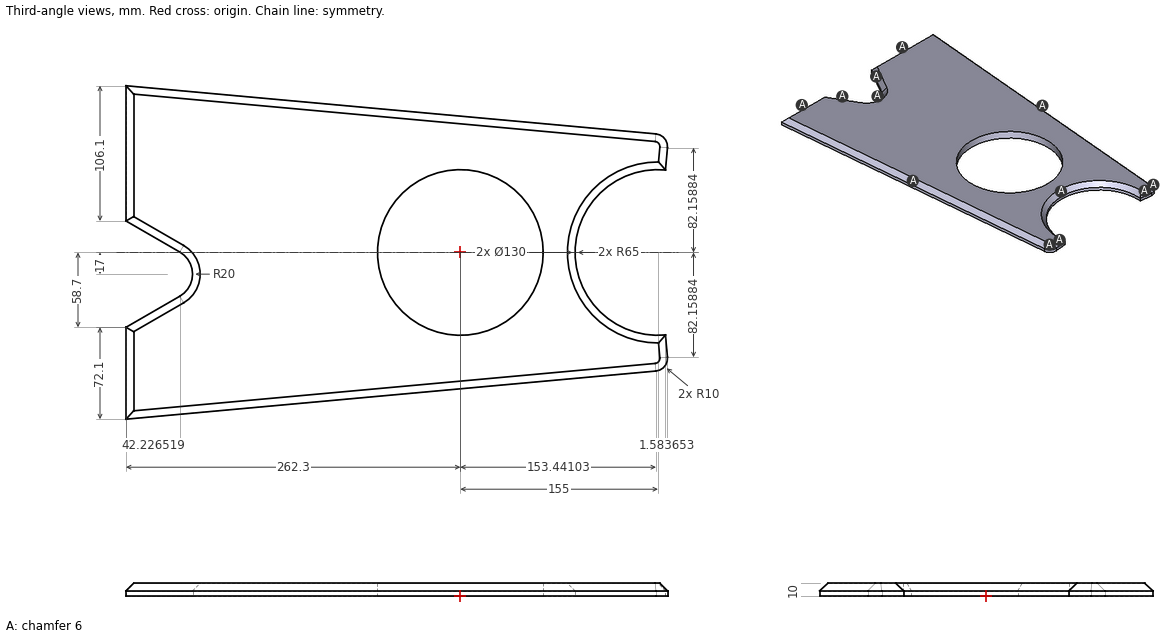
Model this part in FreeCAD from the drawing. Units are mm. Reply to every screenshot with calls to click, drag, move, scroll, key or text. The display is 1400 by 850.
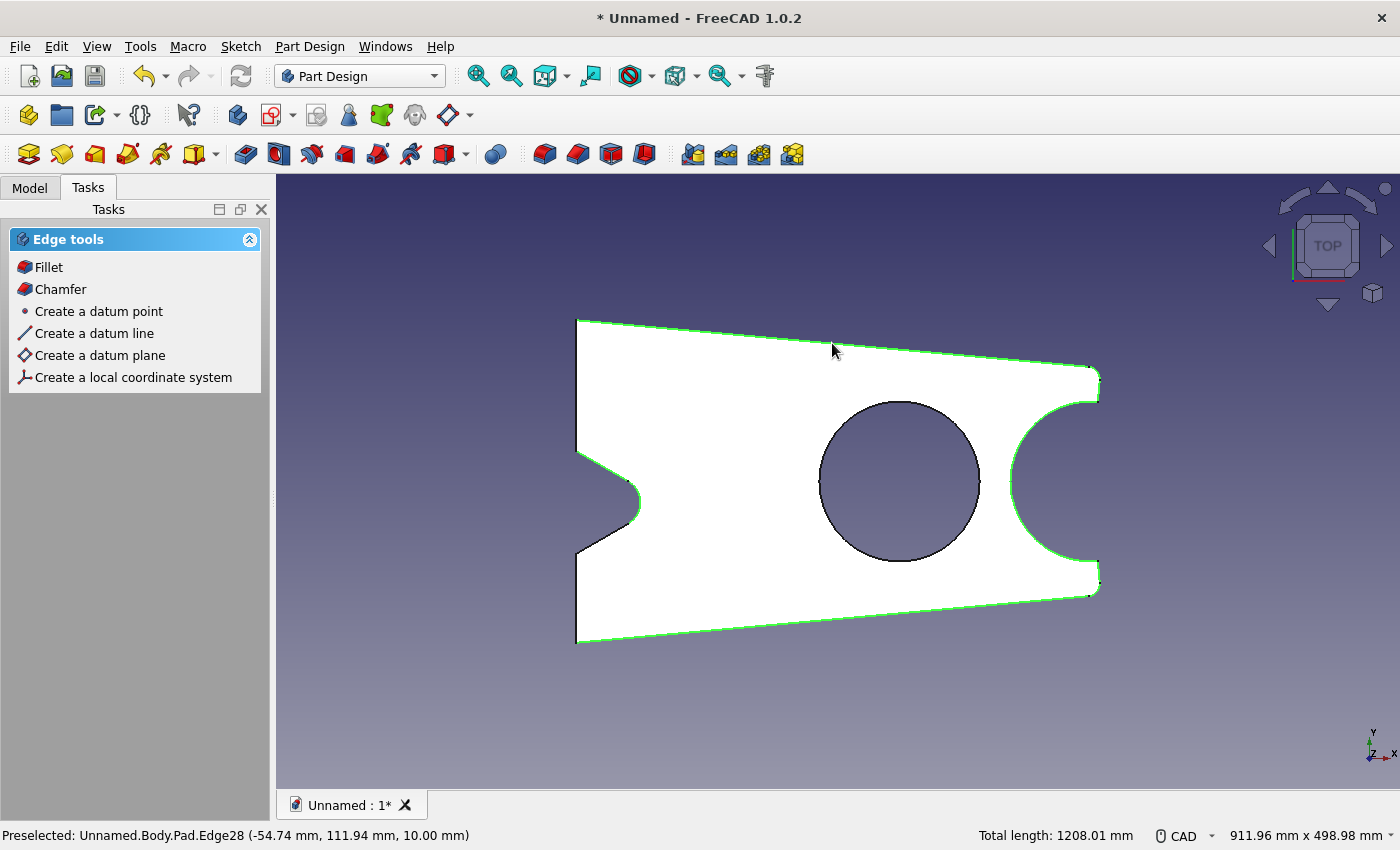
click(576, 385, ctrl)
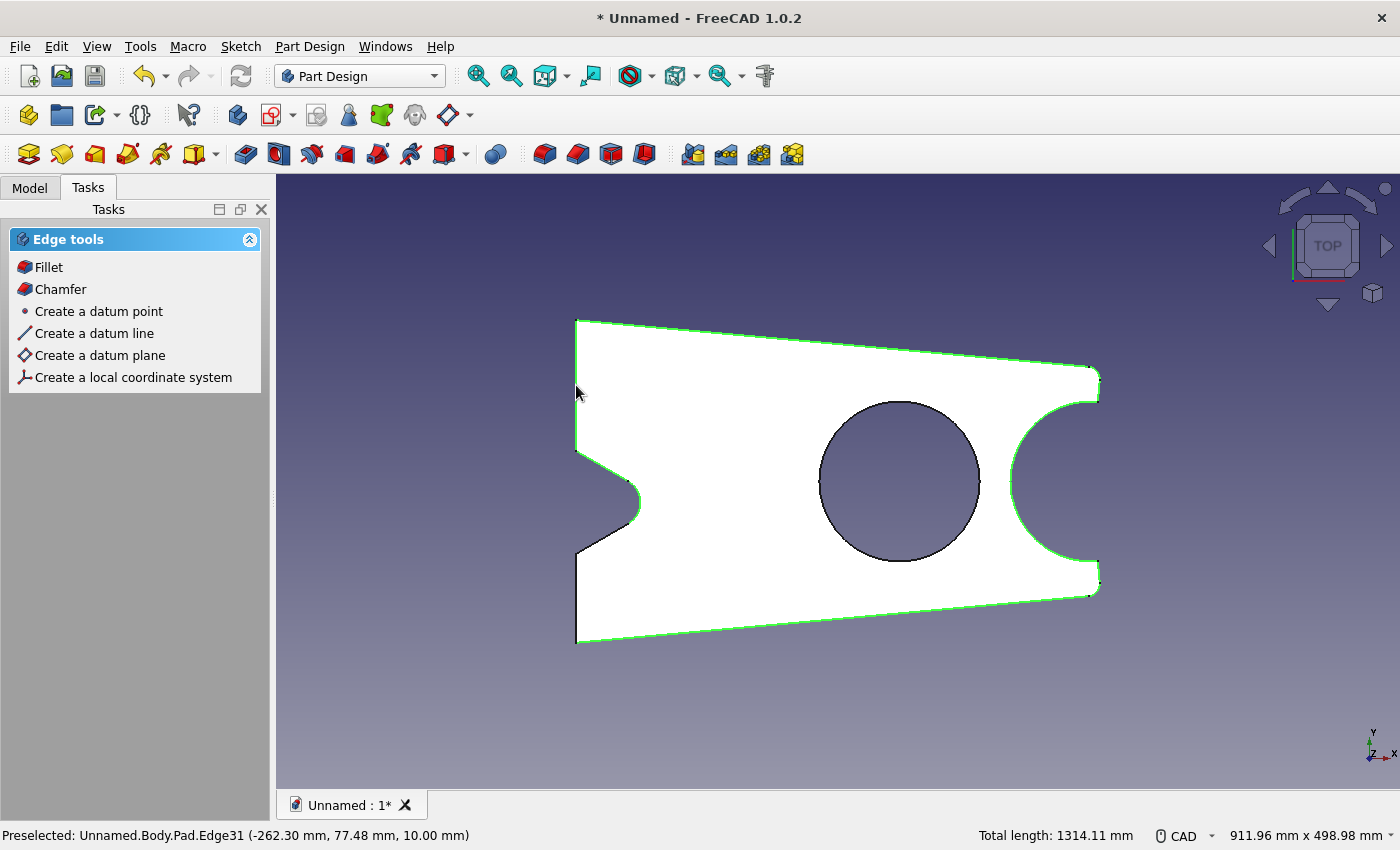
click(602, 538, ctrl)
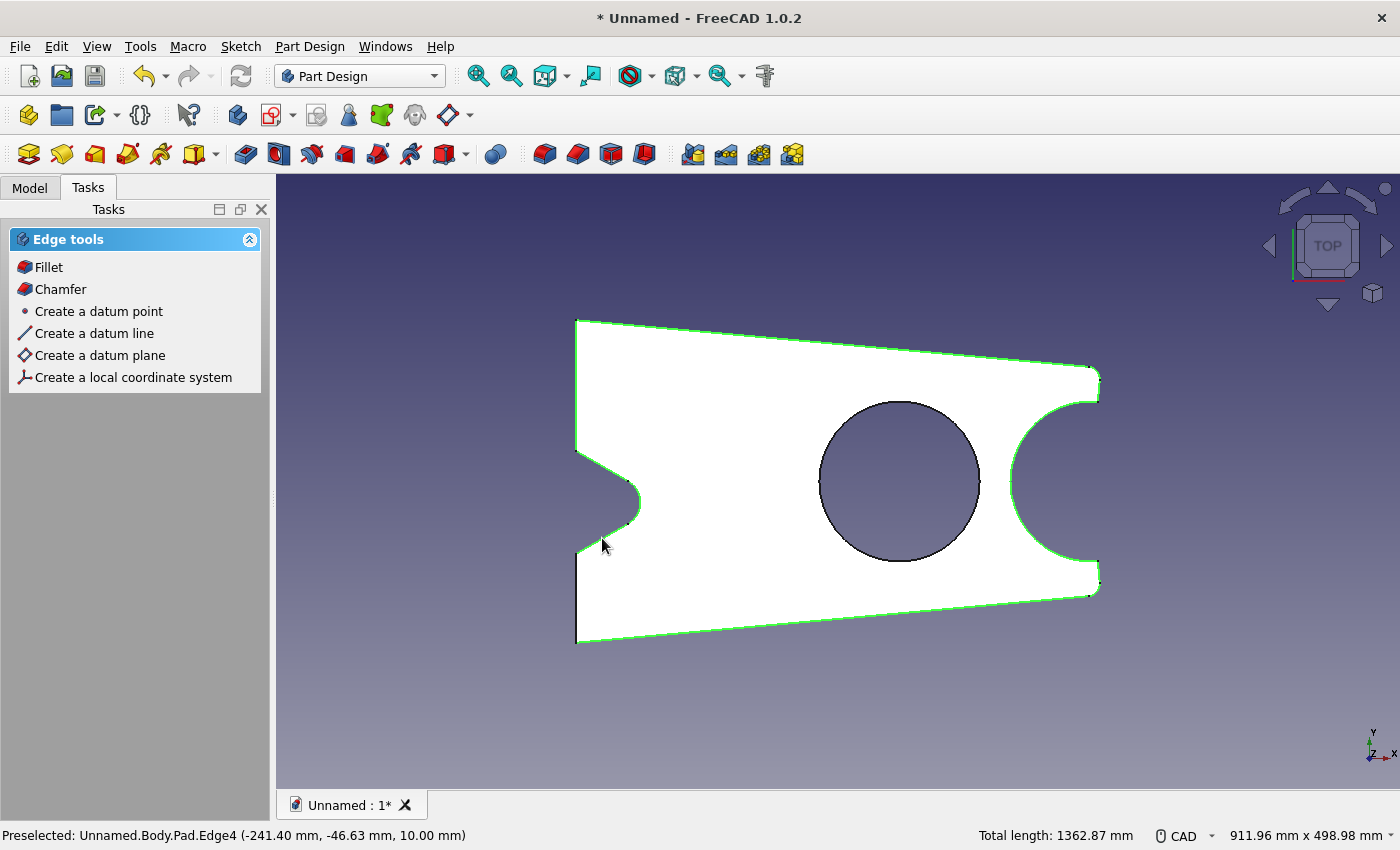
click(576, 597, ctrl)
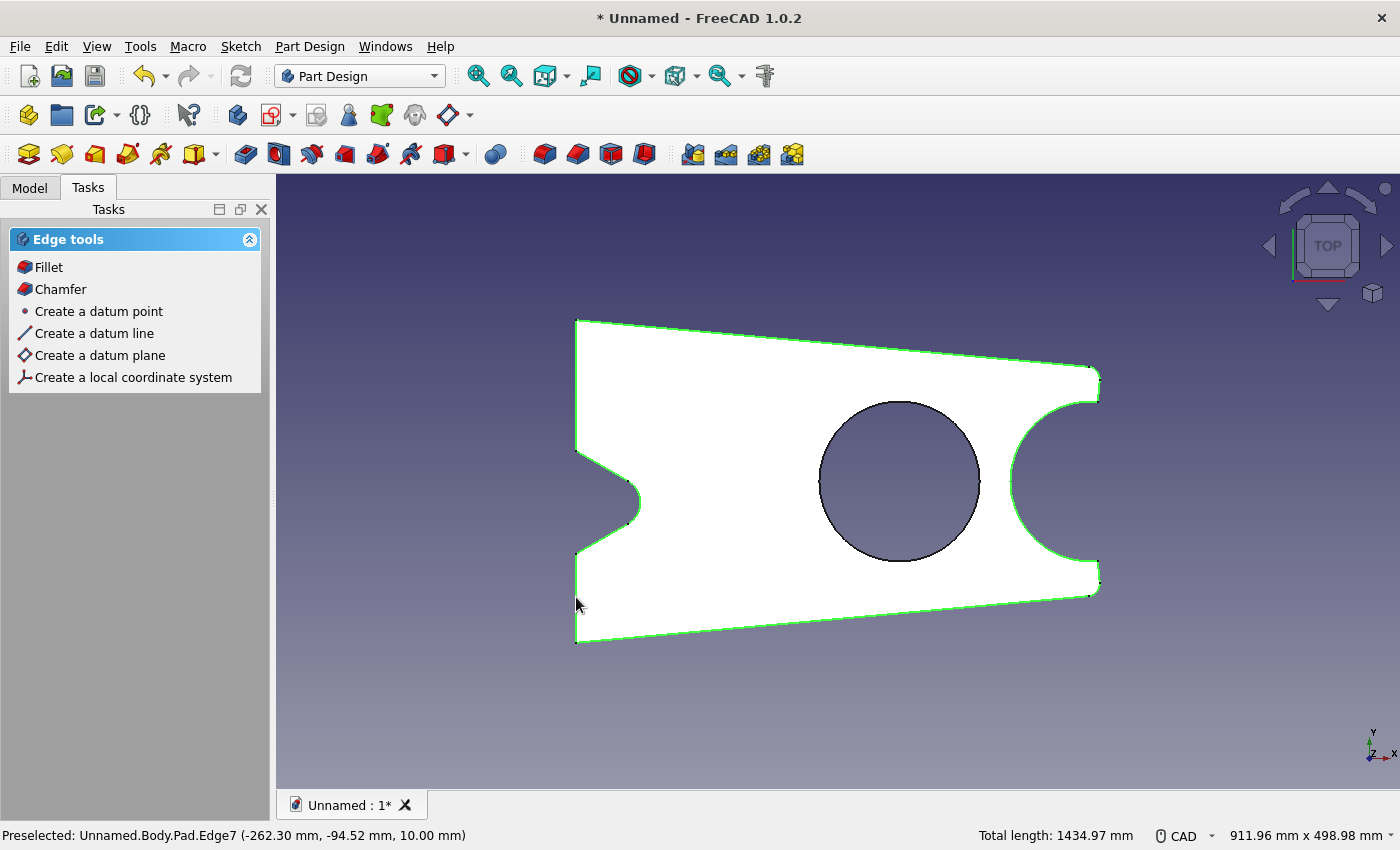
click(578, 154)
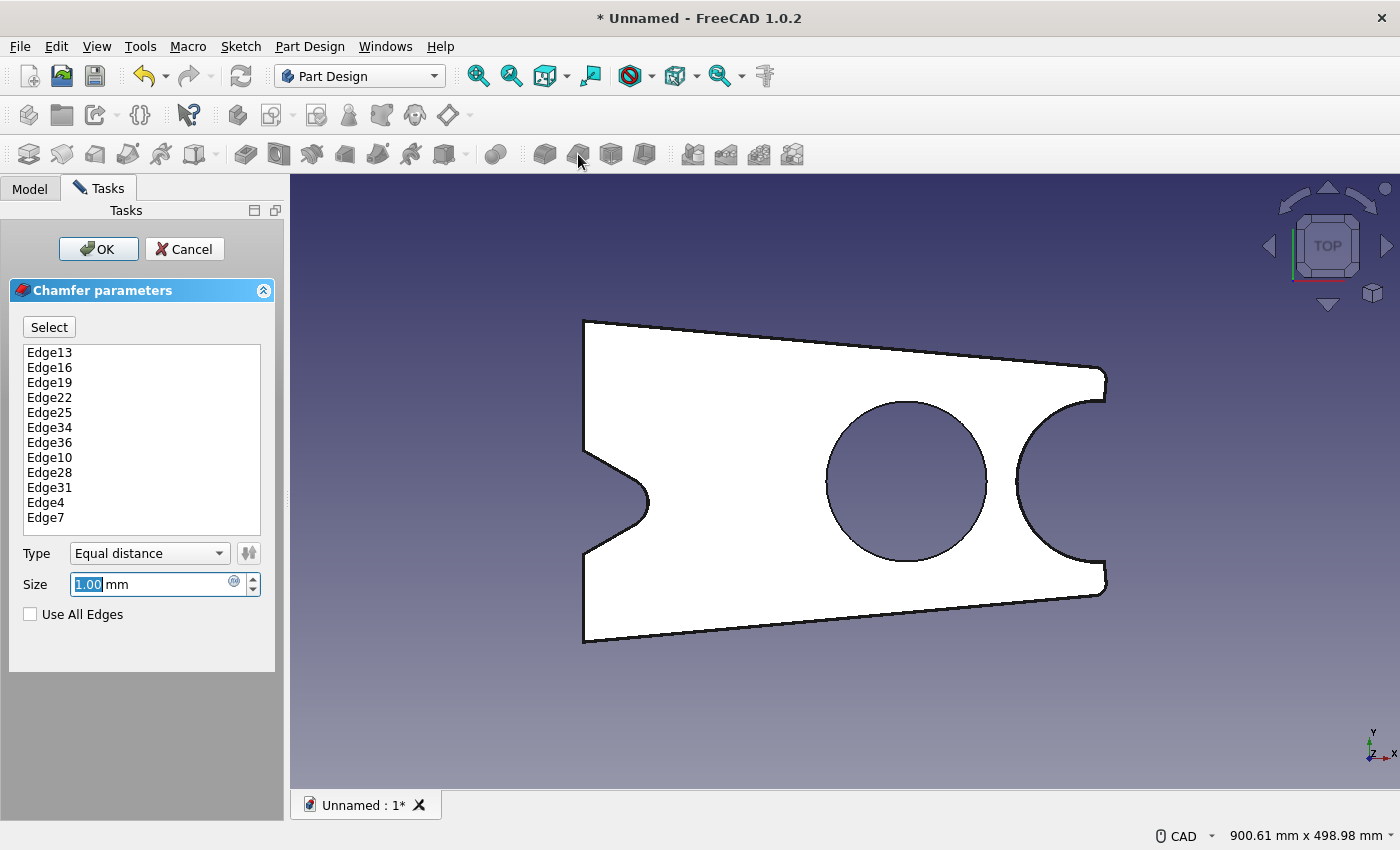
text(6)
key(Tab)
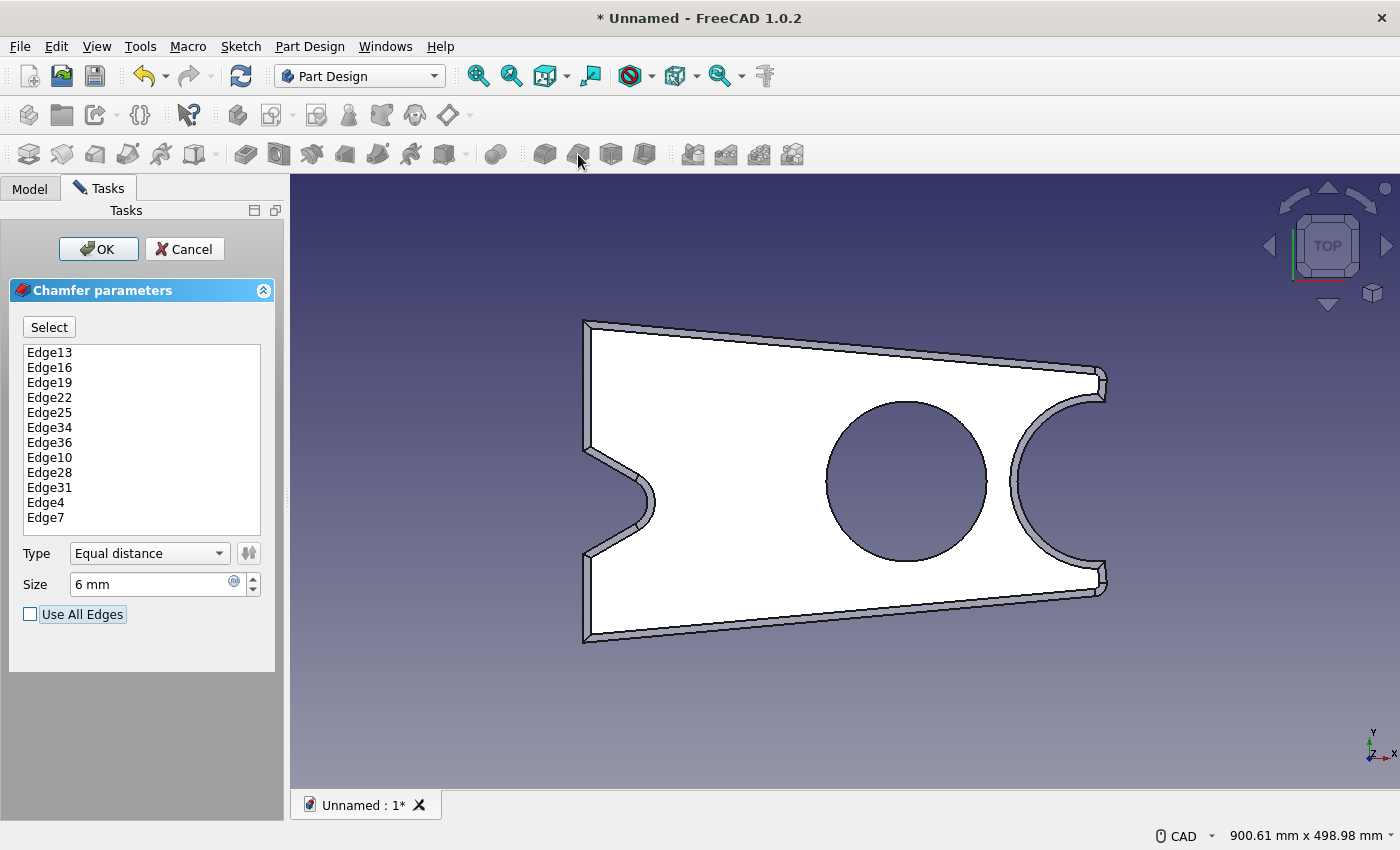
click(99, 249)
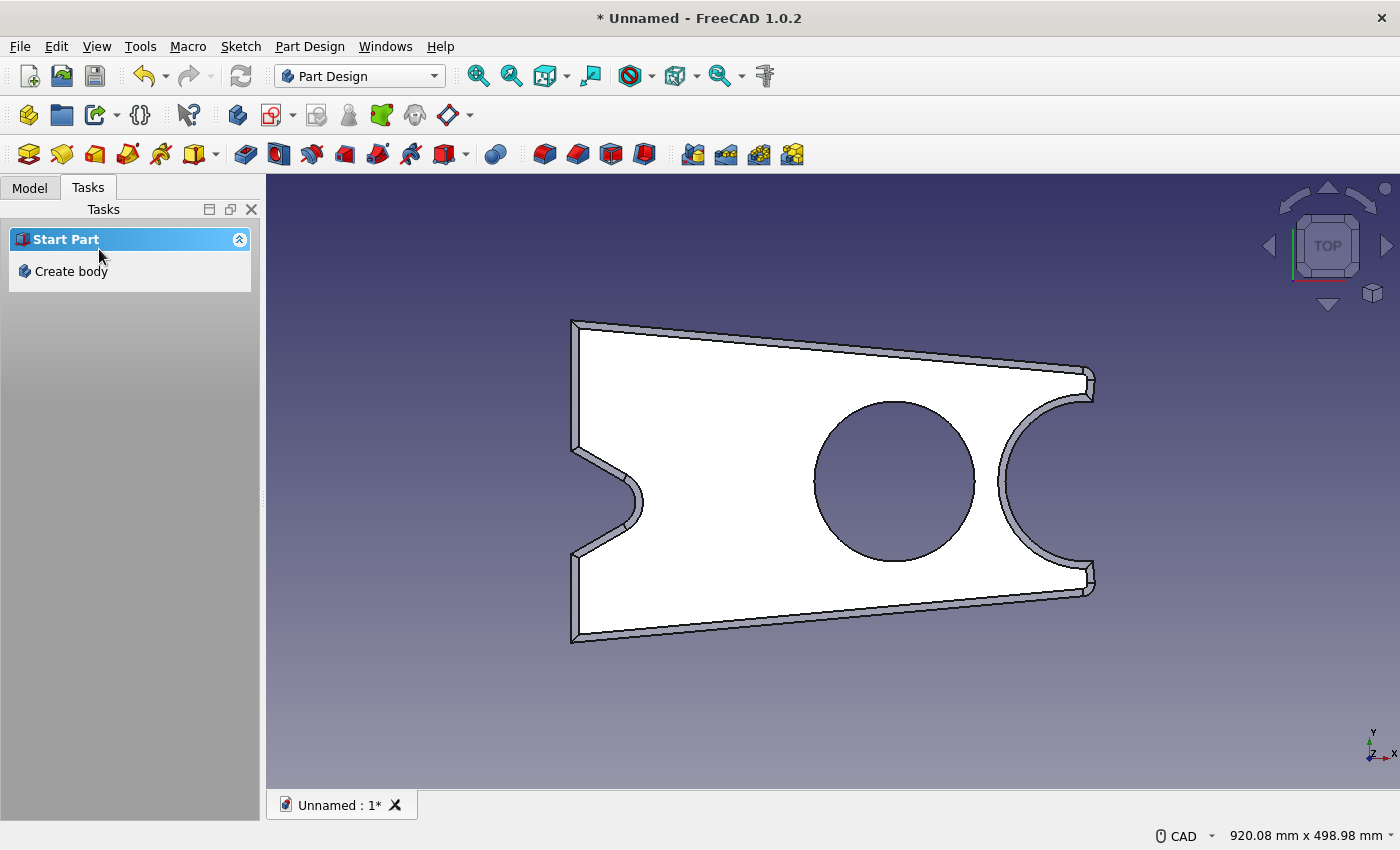
key(0)